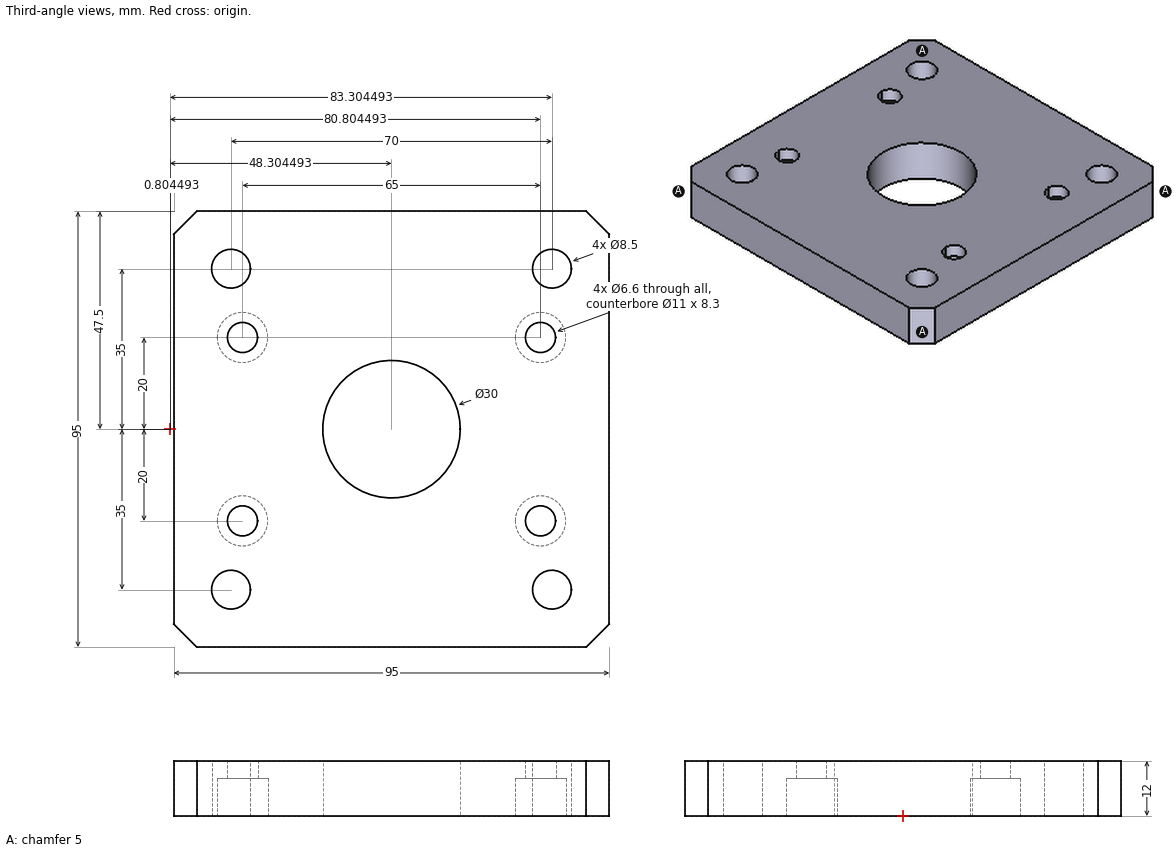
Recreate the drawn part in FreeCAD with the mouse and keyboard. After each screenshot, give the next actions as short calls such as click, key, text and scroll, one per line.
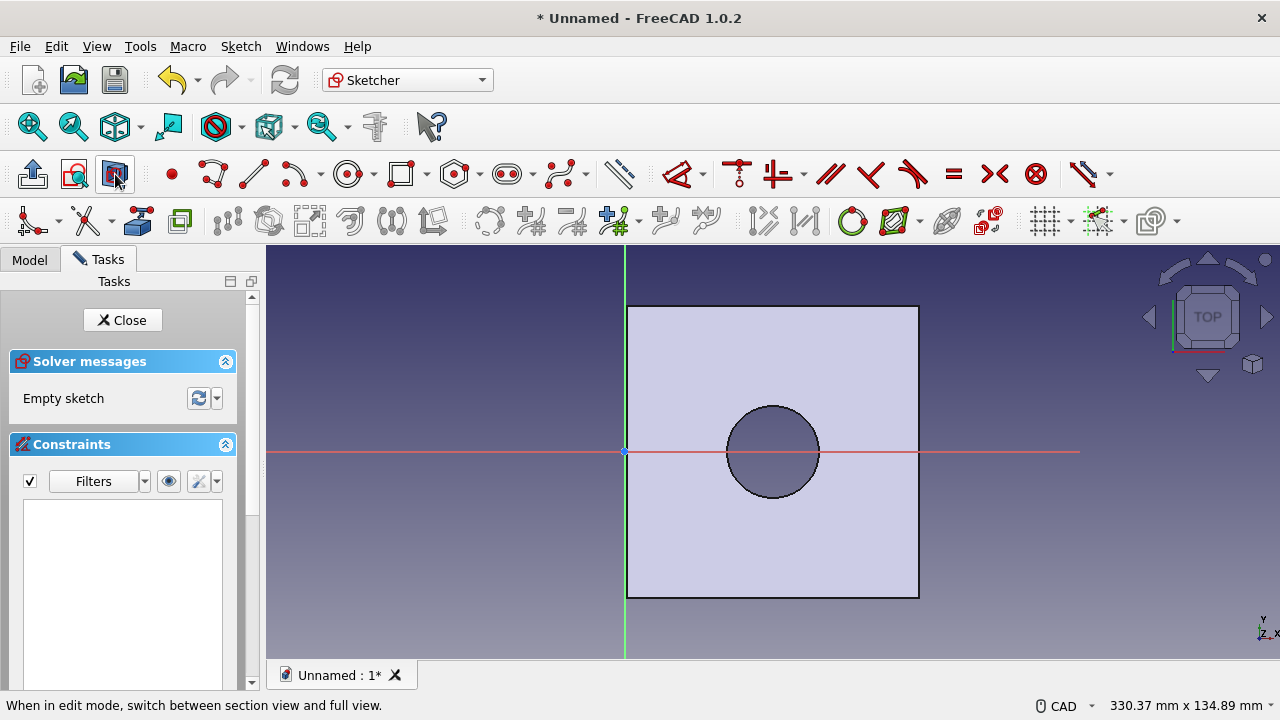
scroll(814, 452, up, 3)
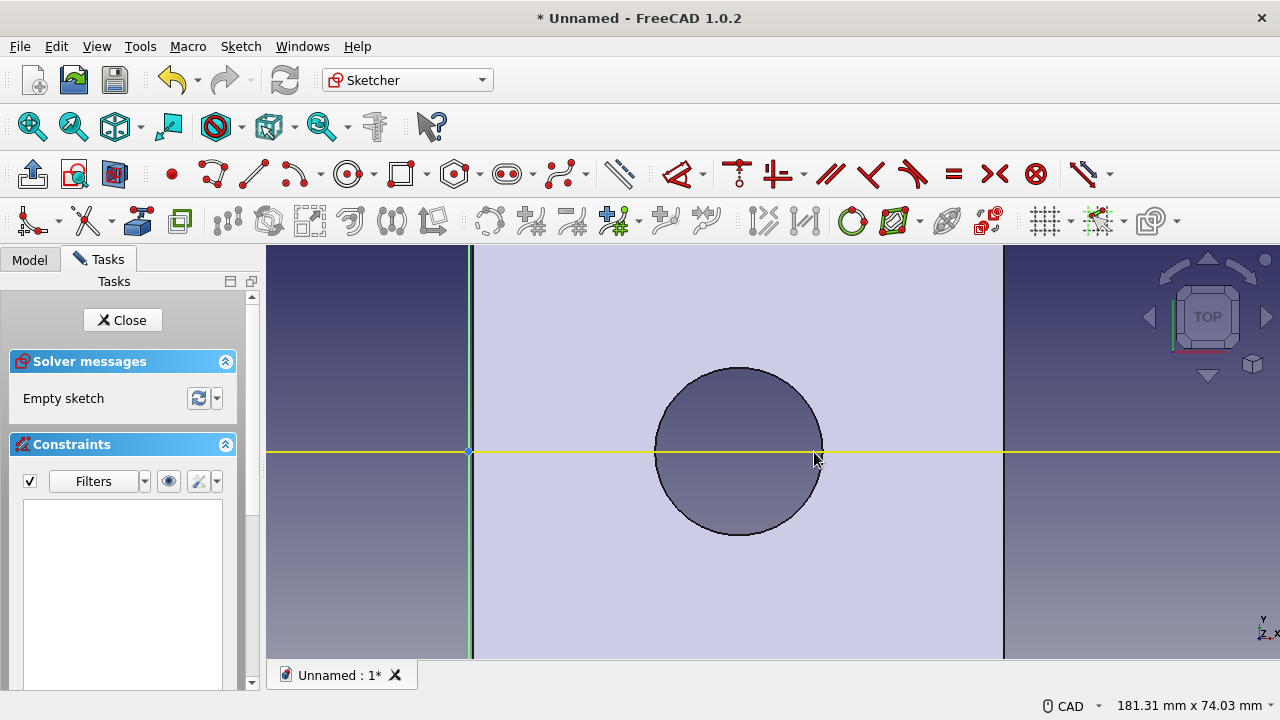
click(348, 174)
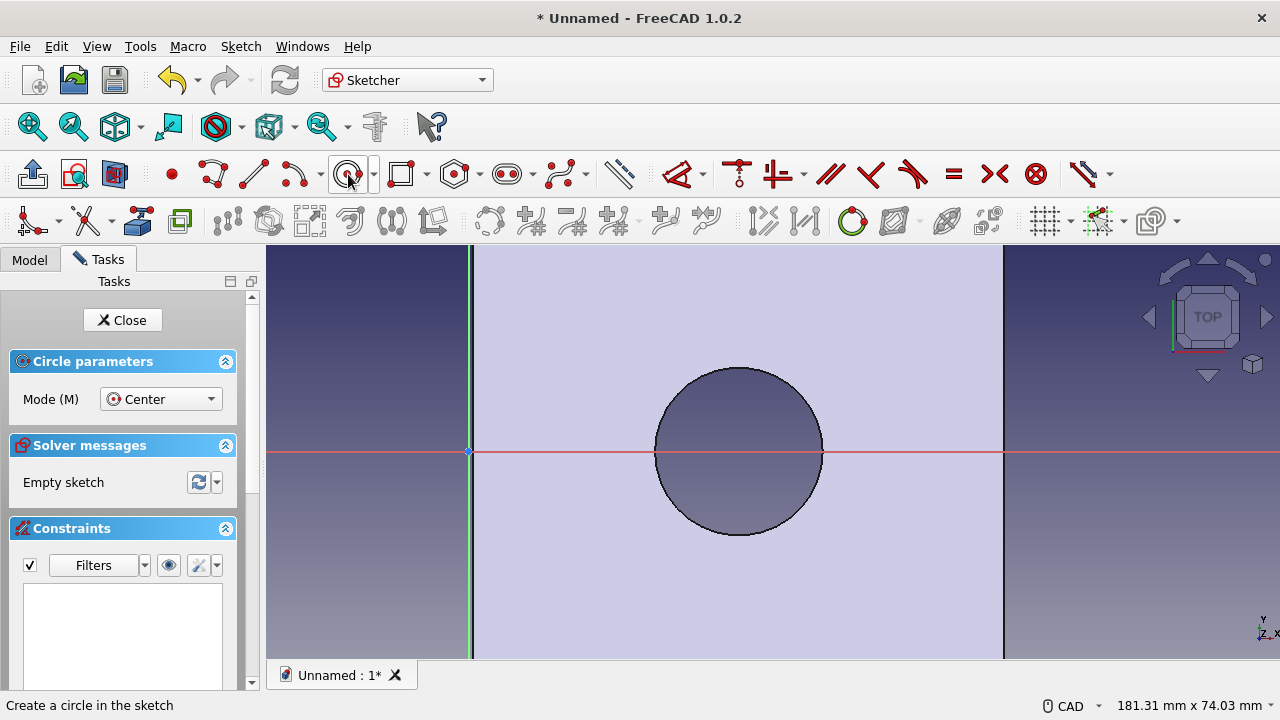
scroll(921, 340, up, 2)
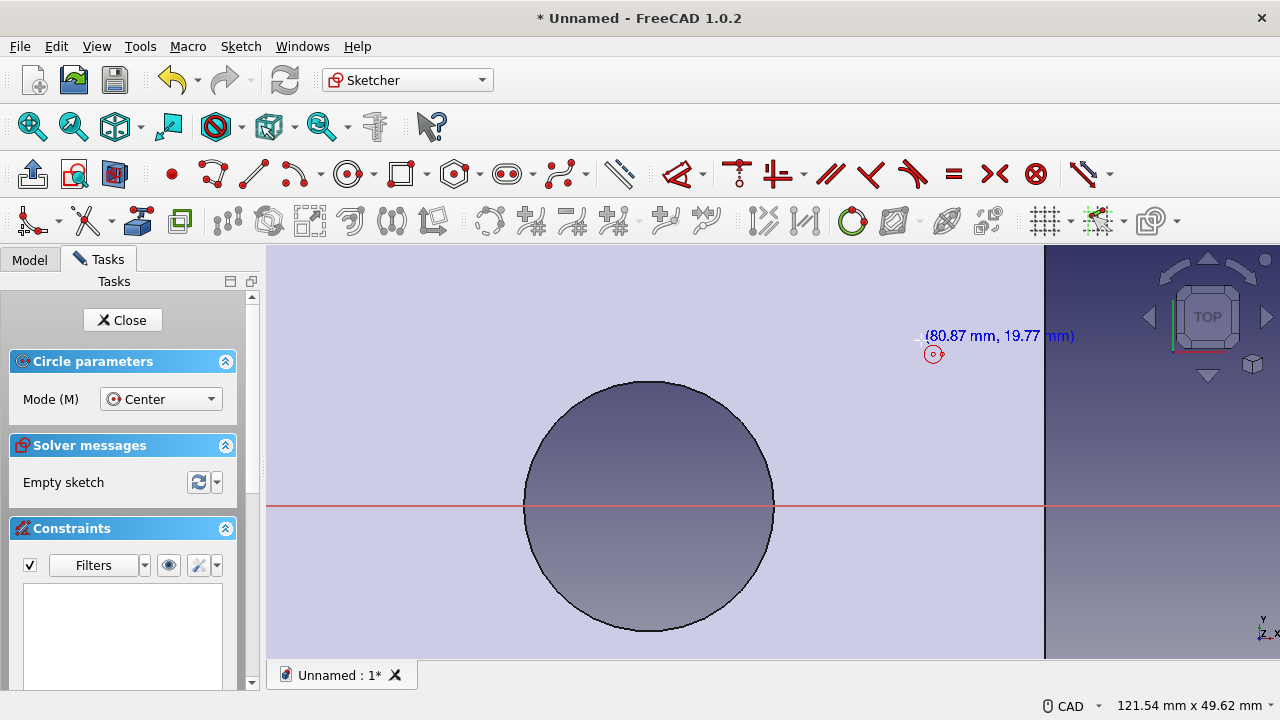
click(920, 339)
click(940, 320)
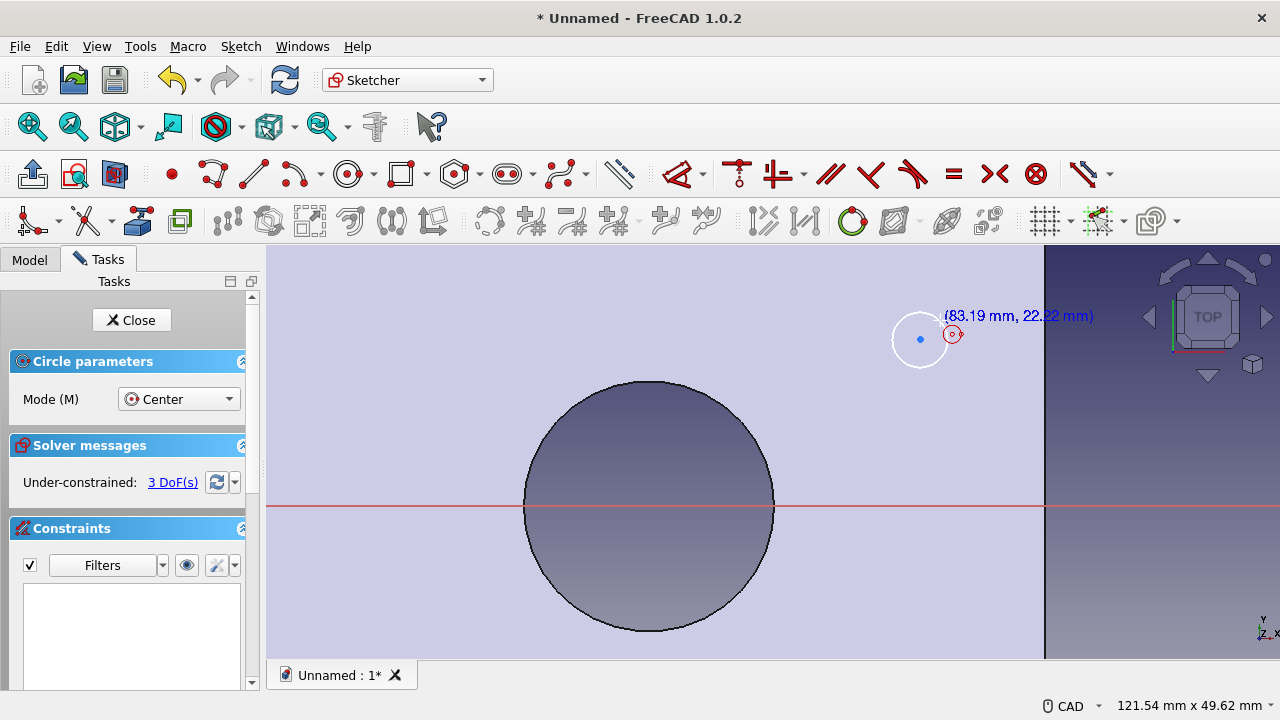
click(378, 339)
click(397, 320)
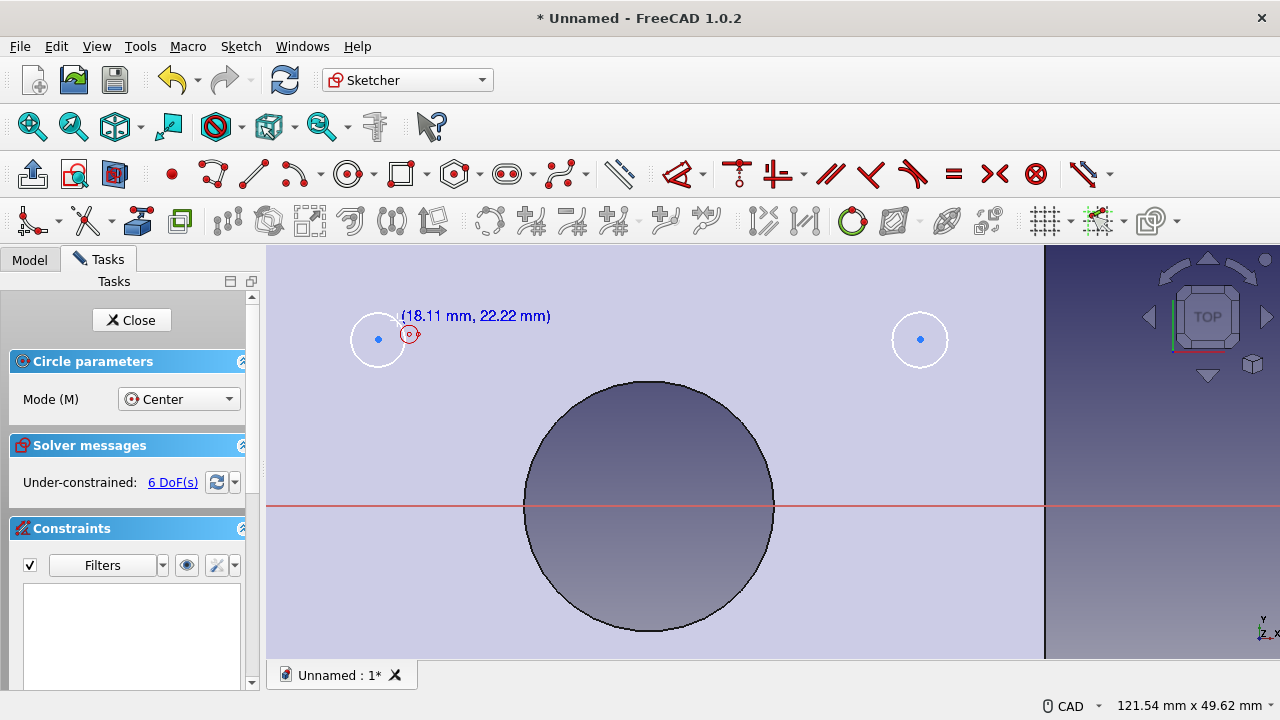
scroll(924, 341, down, 2)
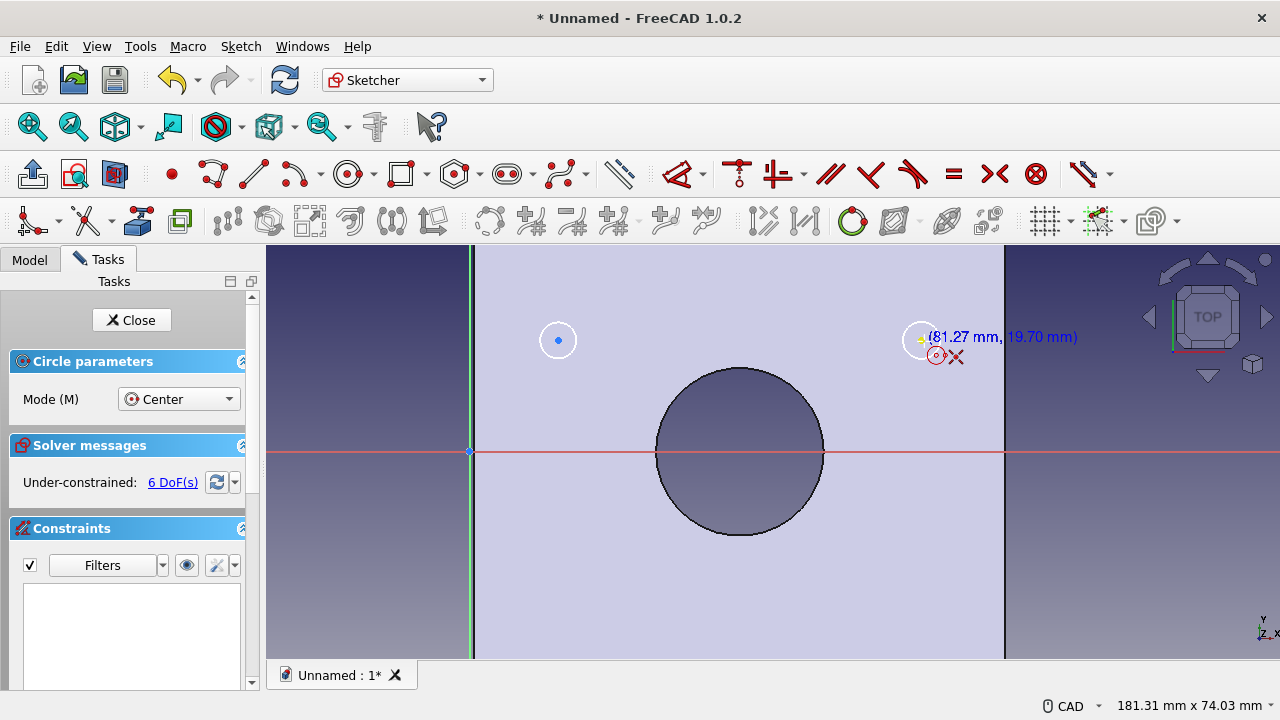
scroll(558, 564, up, 2)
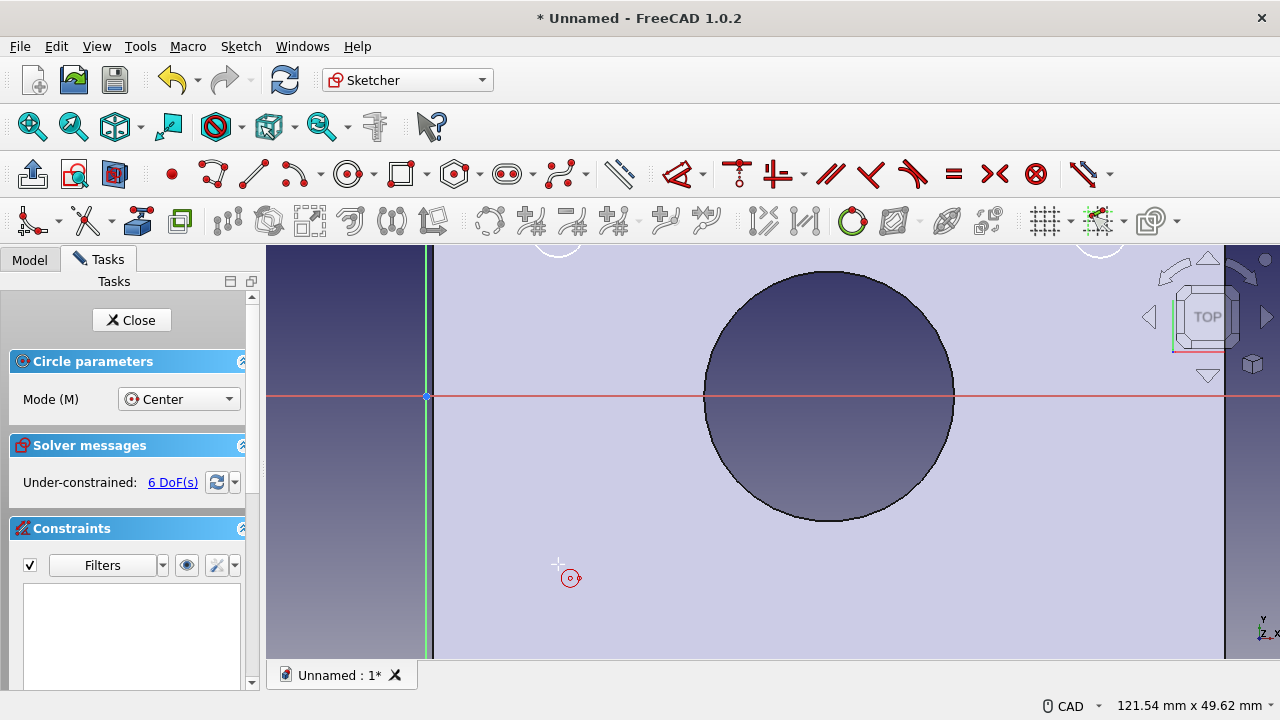
click(558, 563)
click(577, 544)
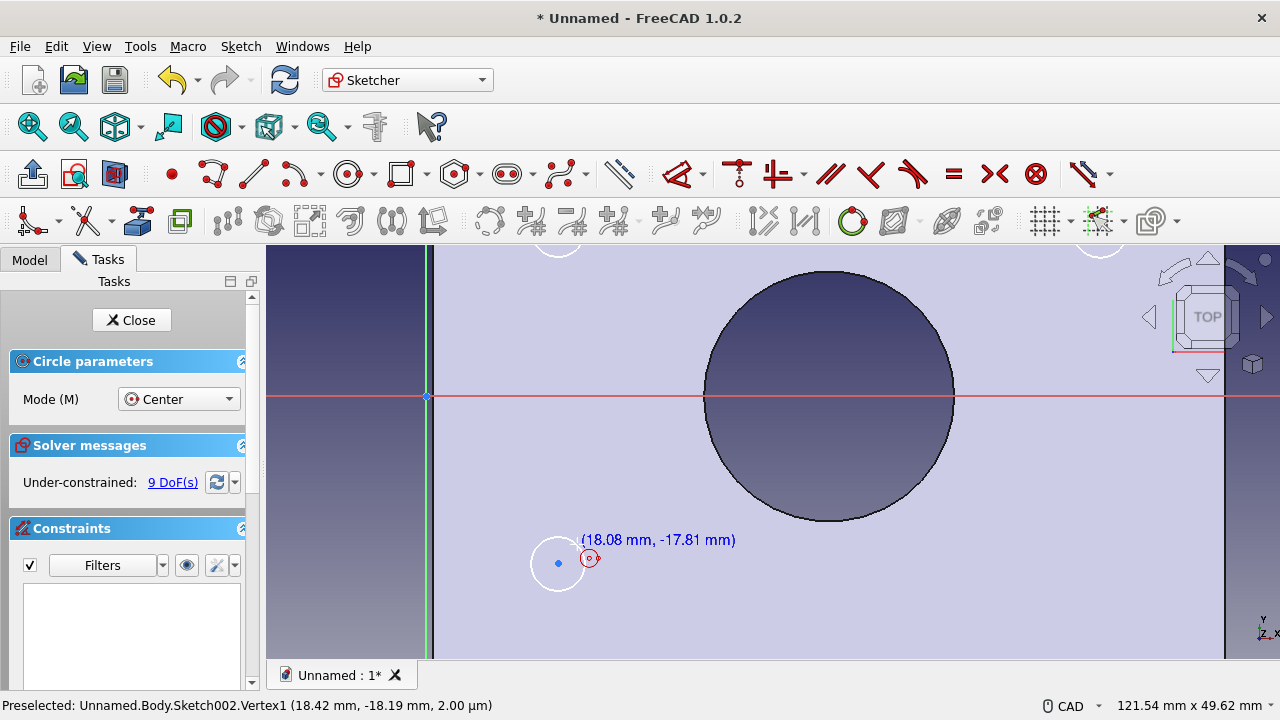
click(1100, 563)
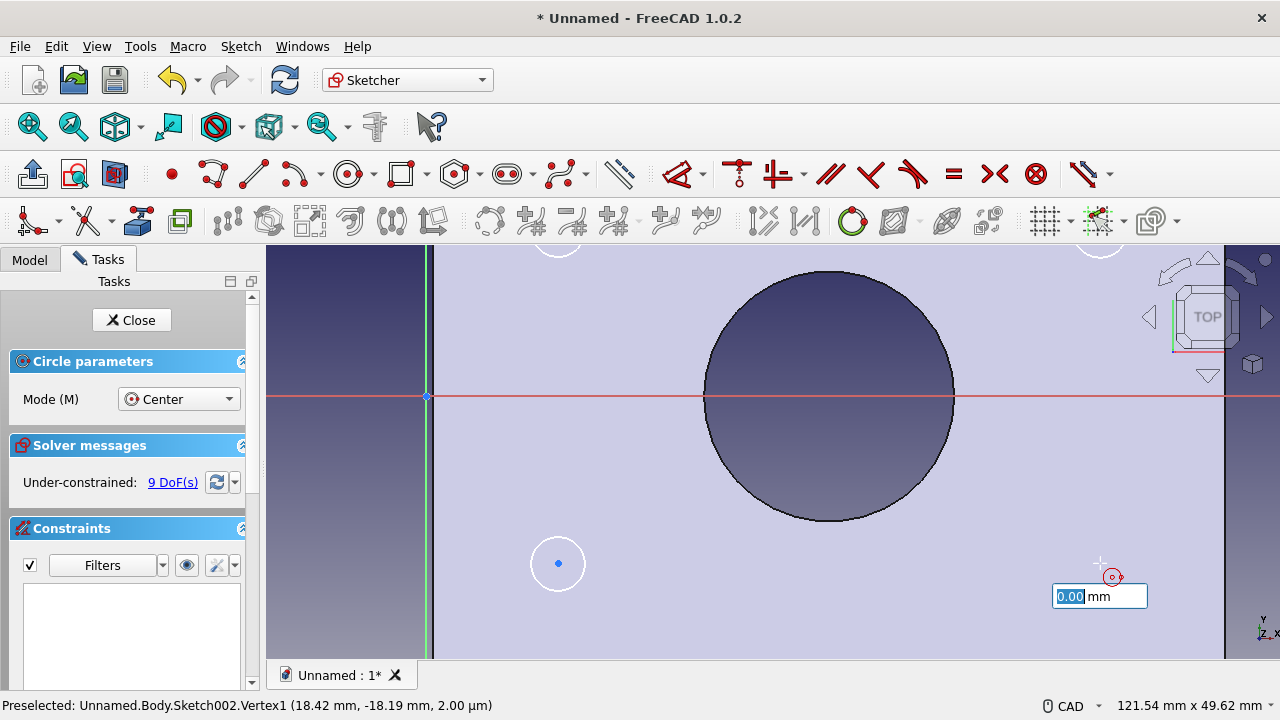
scroll(557, 565, down, 2)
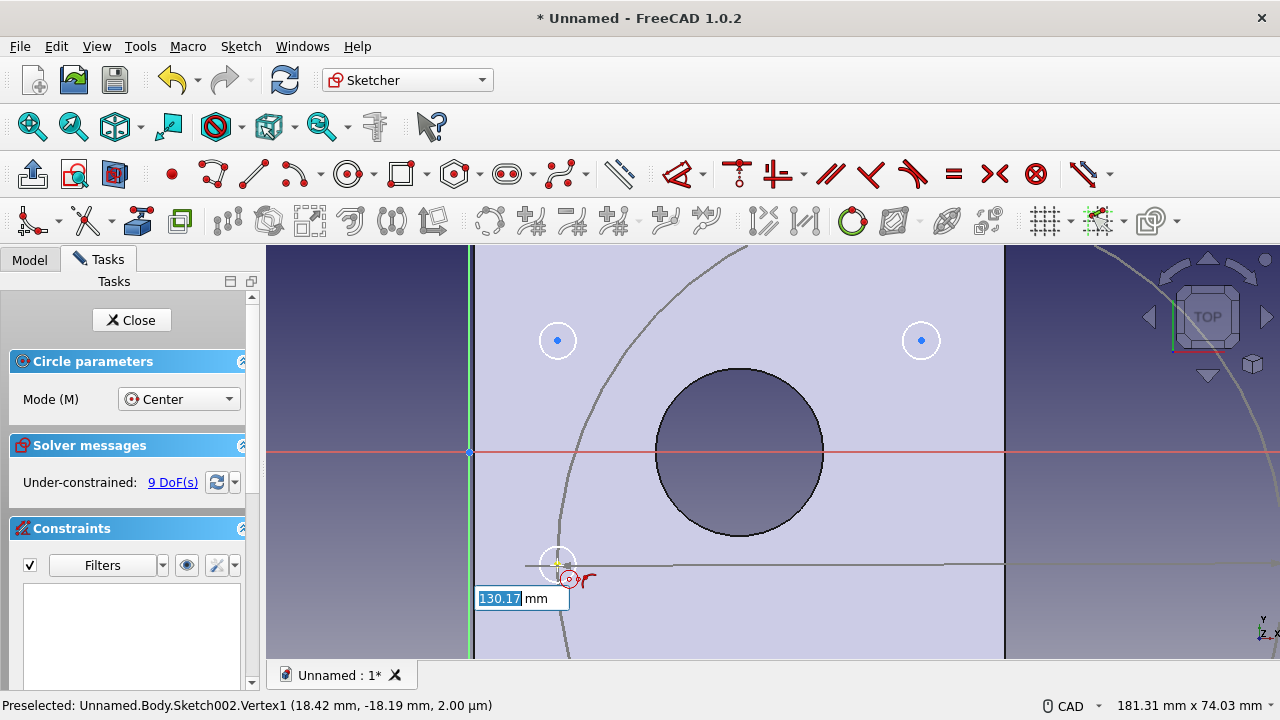
click(934, 551)
key(Escape)